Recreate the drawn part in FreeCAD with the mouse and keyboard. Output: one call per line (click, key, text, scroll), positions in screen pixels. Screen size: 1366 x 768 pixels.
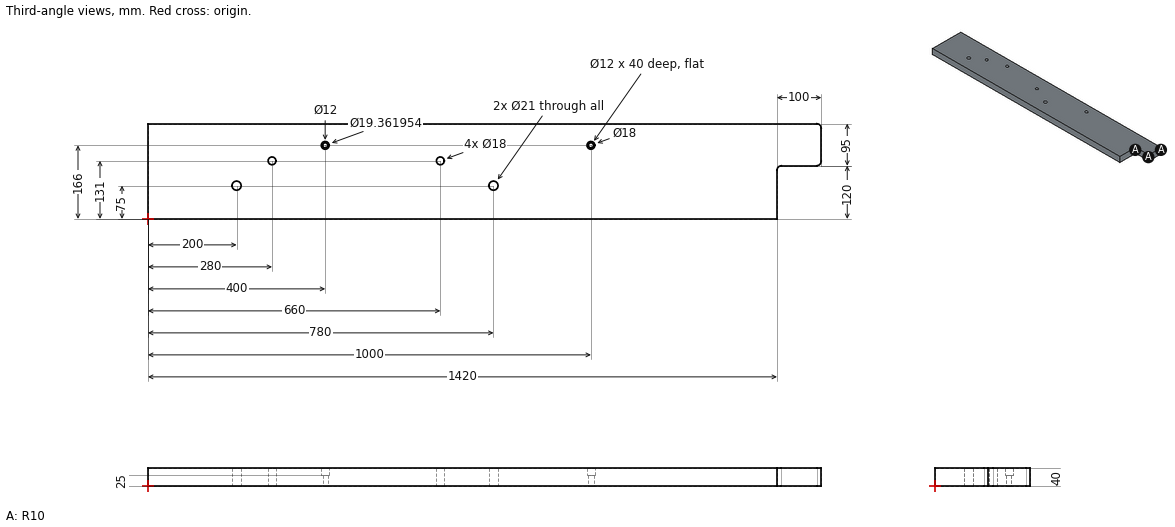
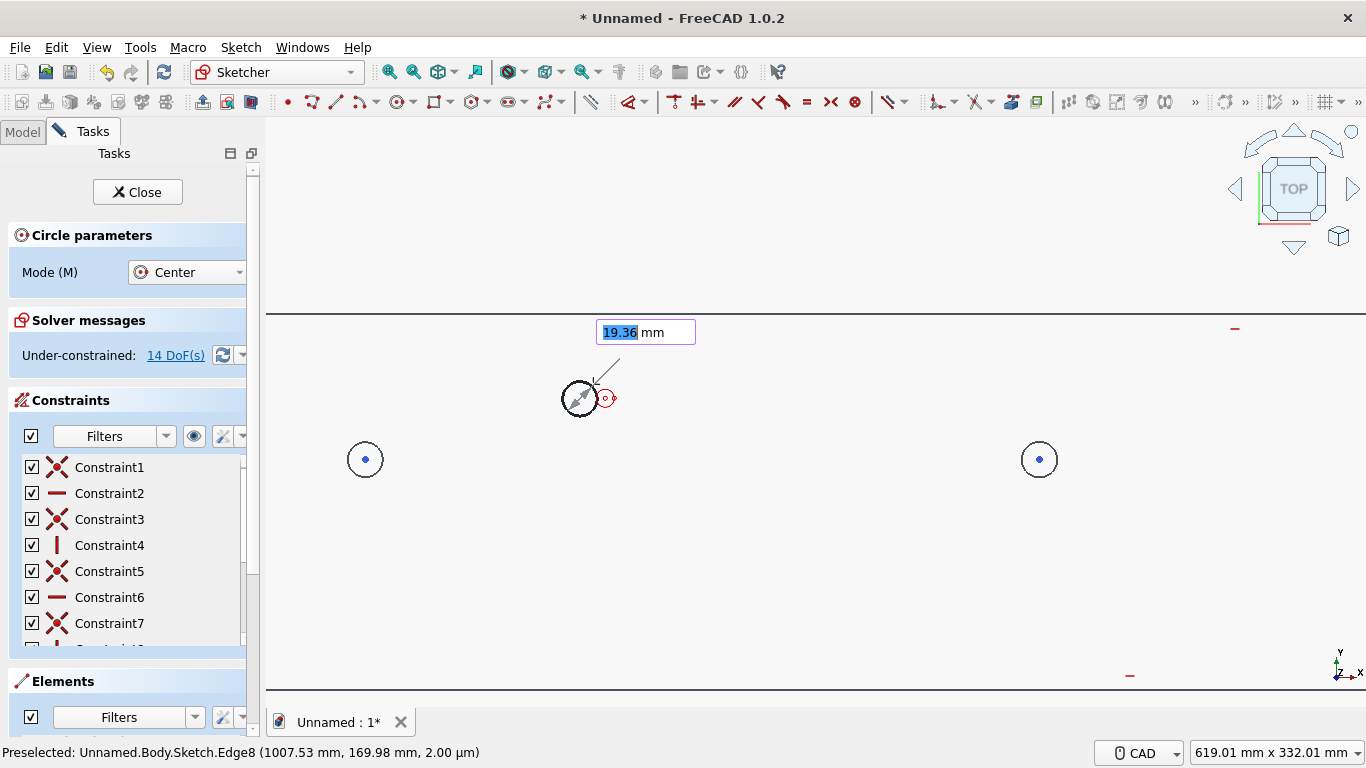
click(590, 384)
key(Escape)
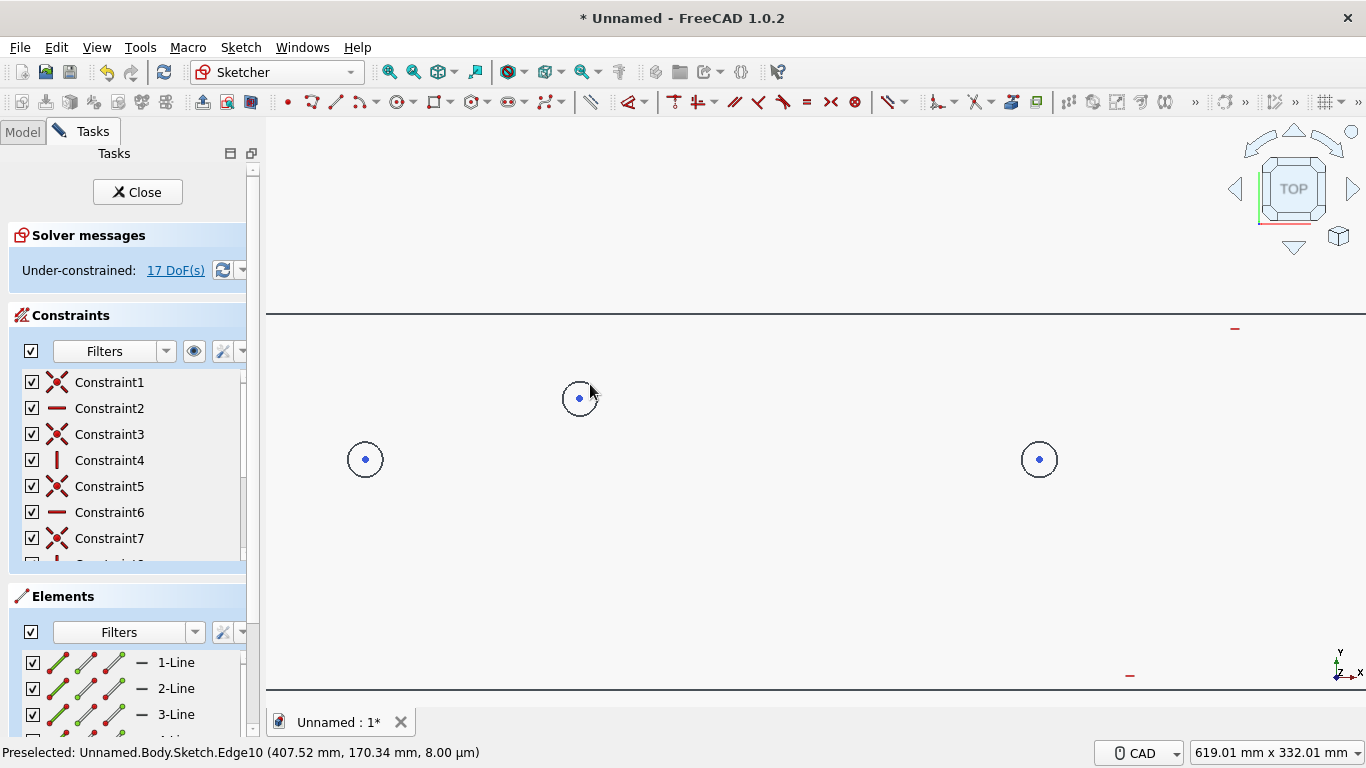
scroll(593, 384, down, 7)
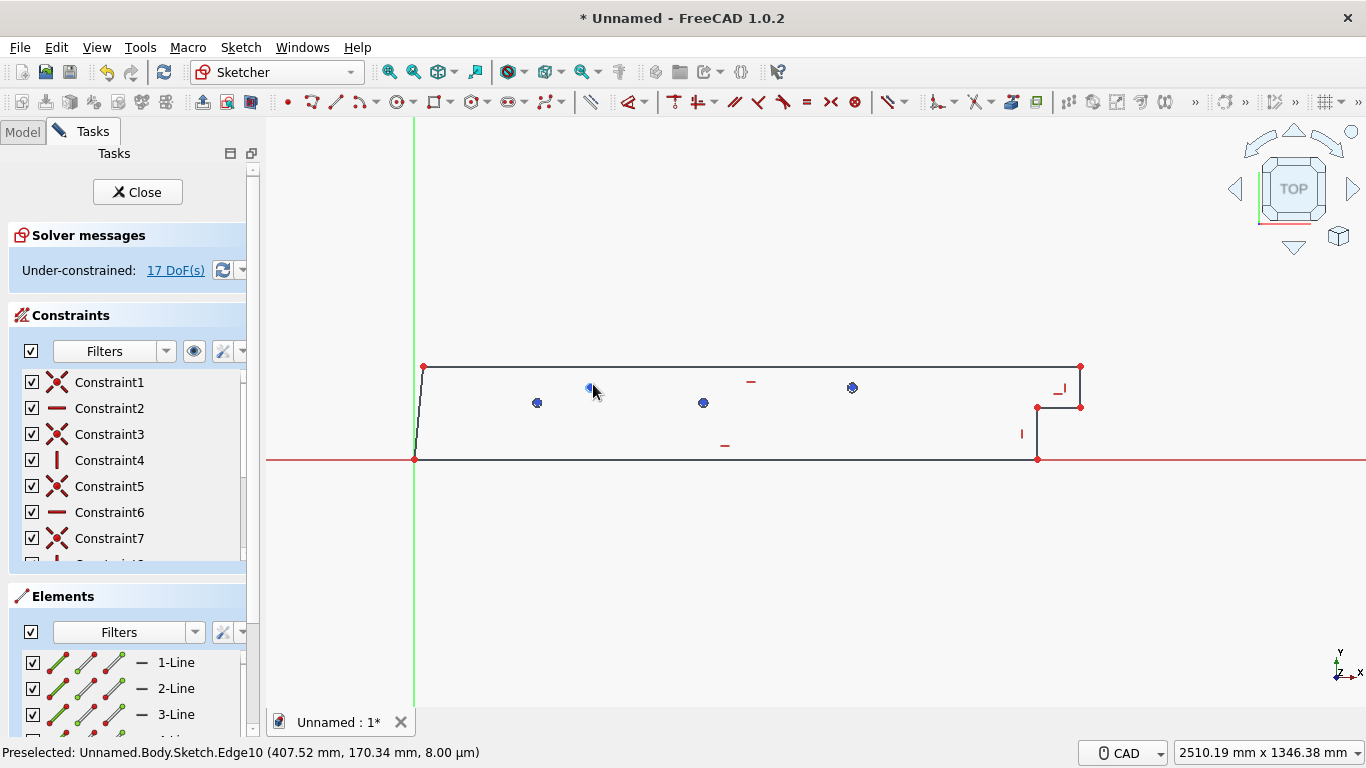
scroll(421, 395, up, 5)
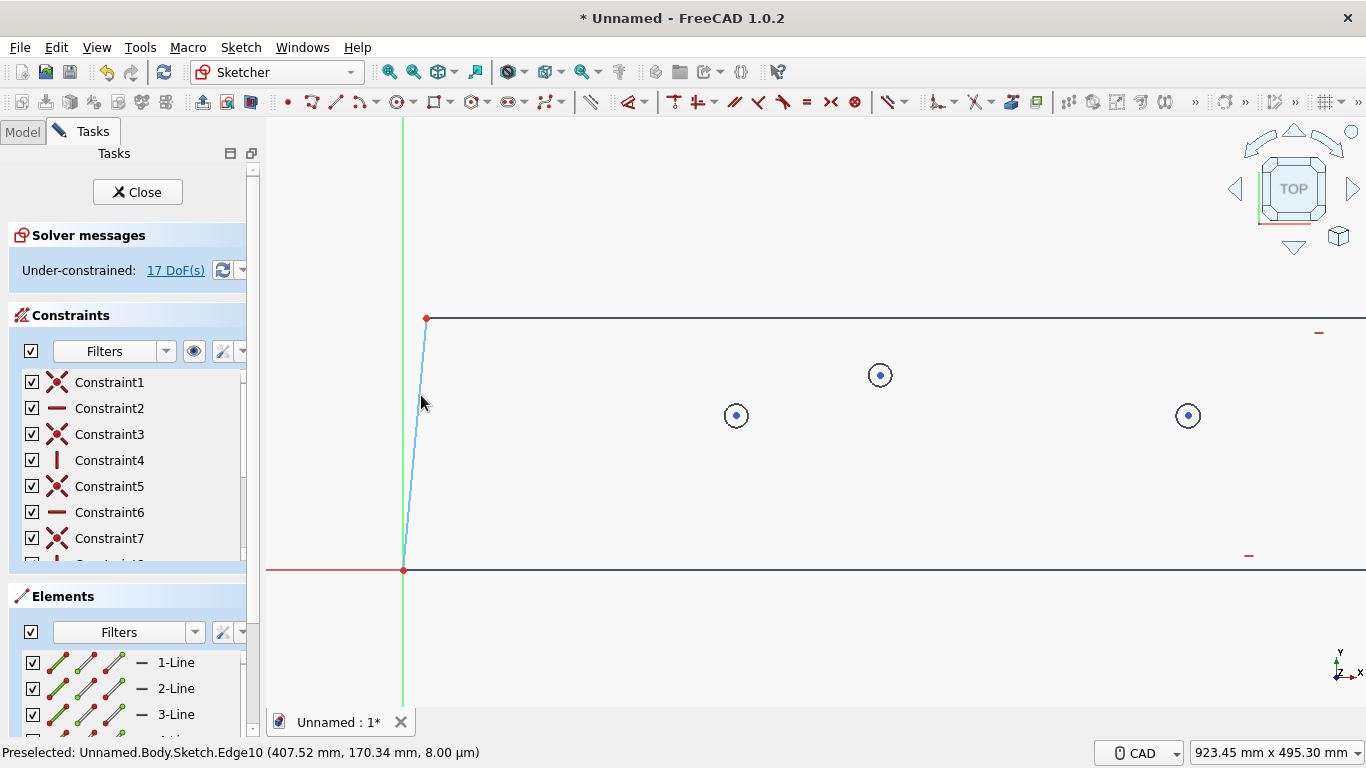
click(420, 394)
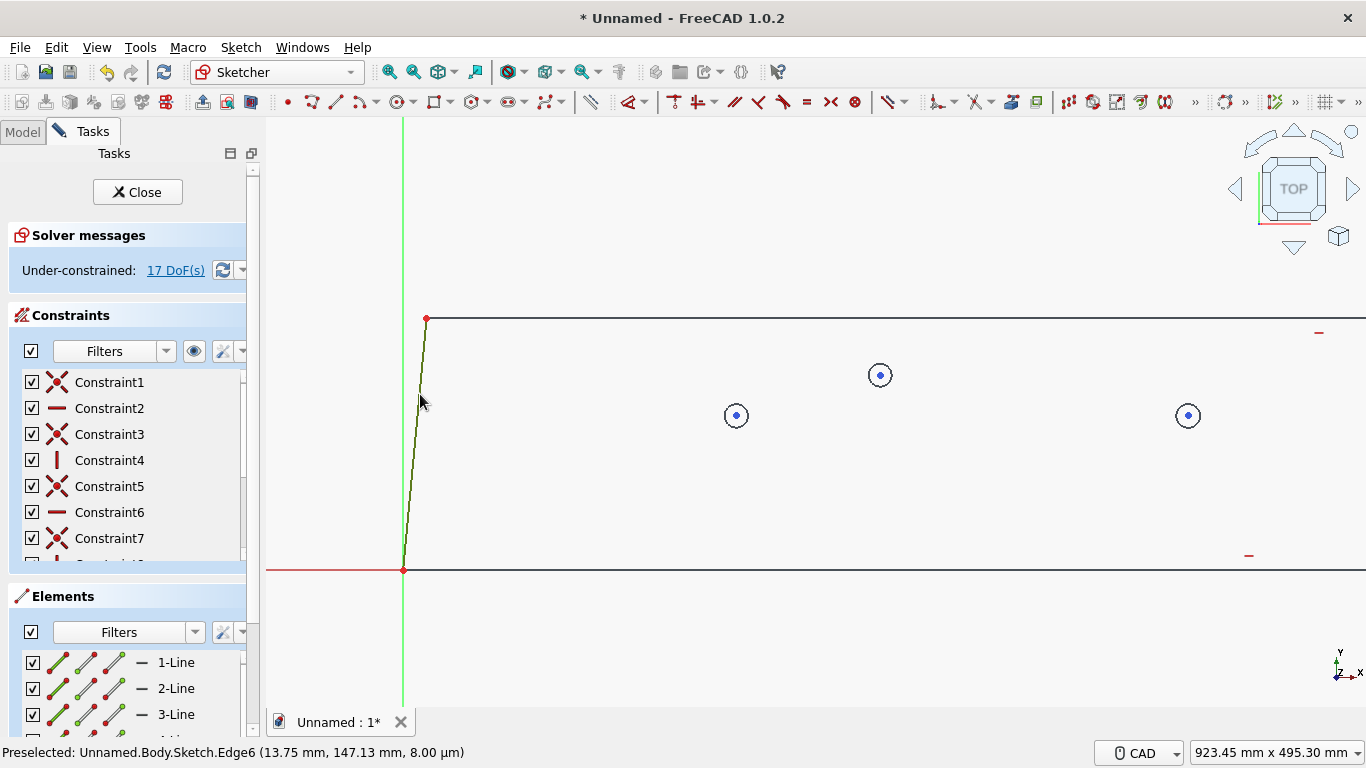
key(v)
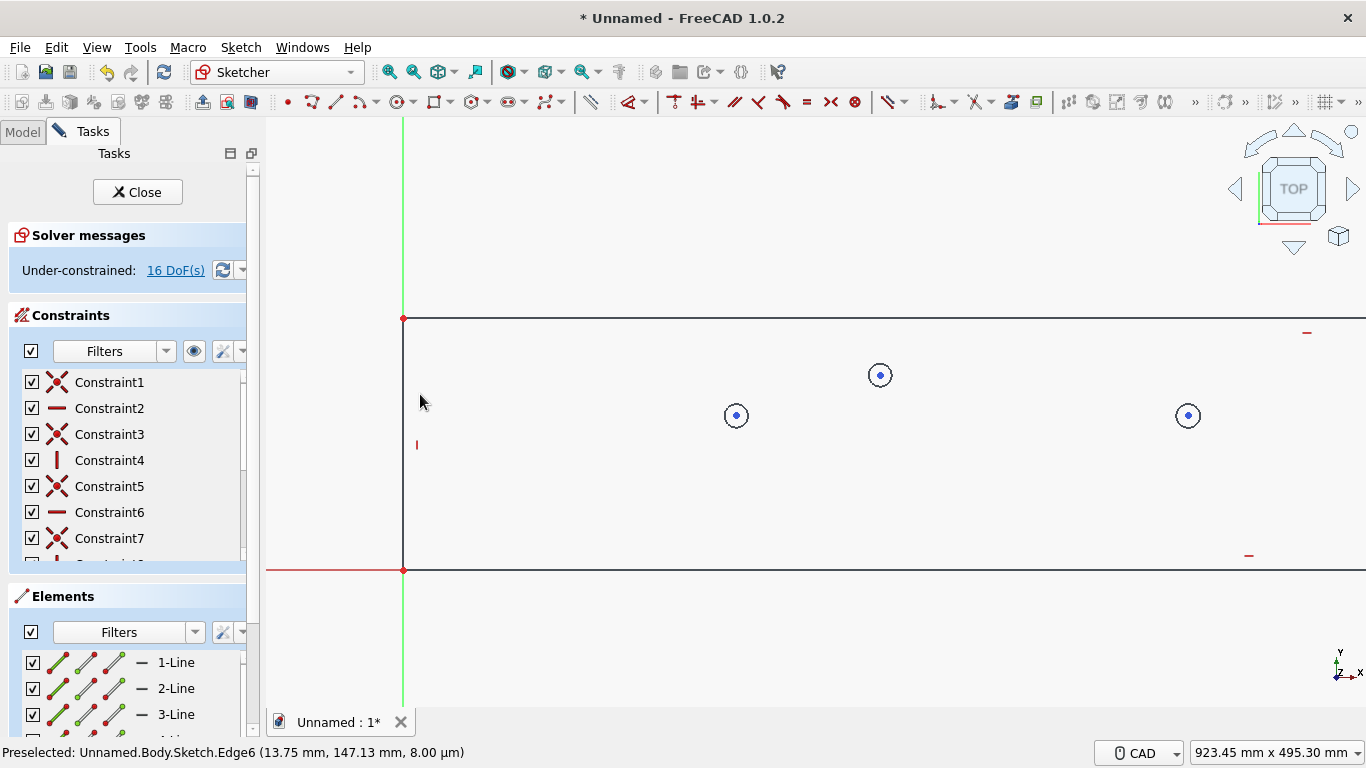
click(1197, 407)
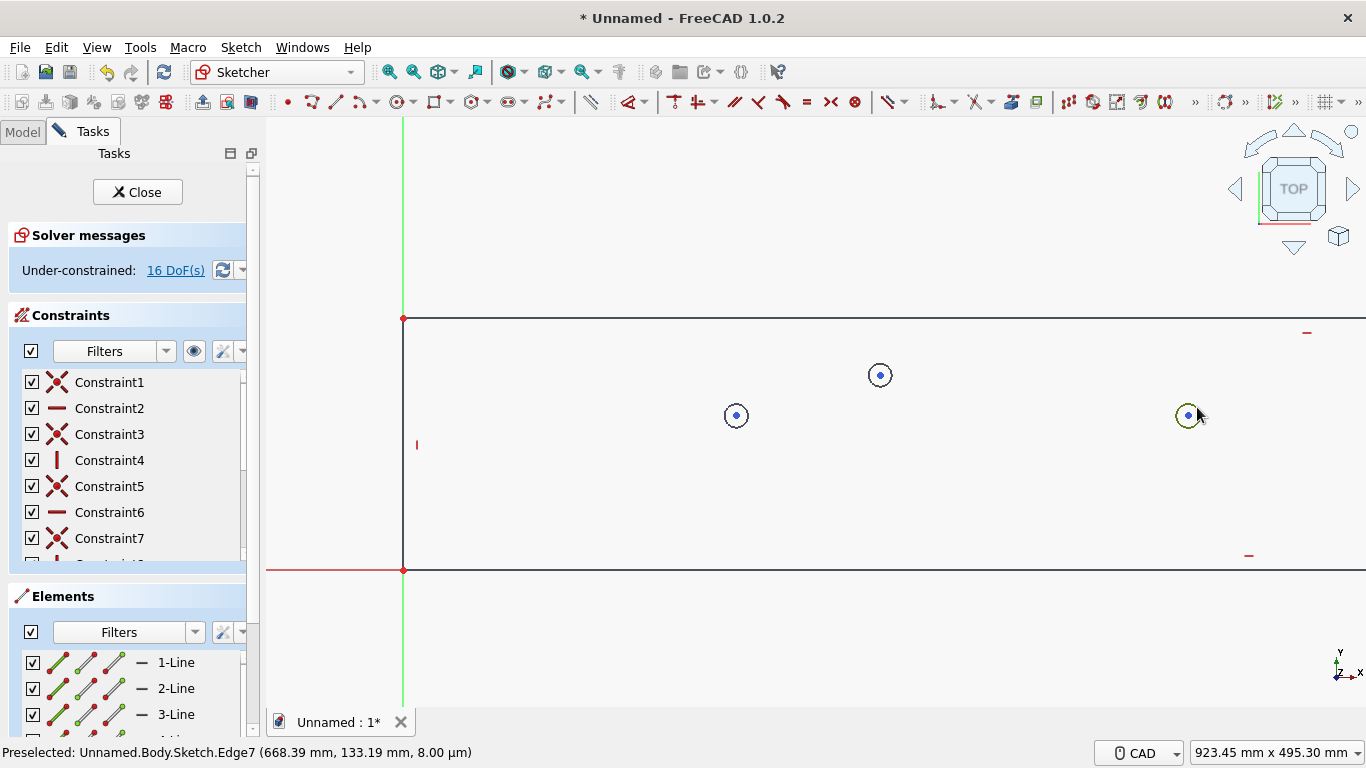
click(745, 408)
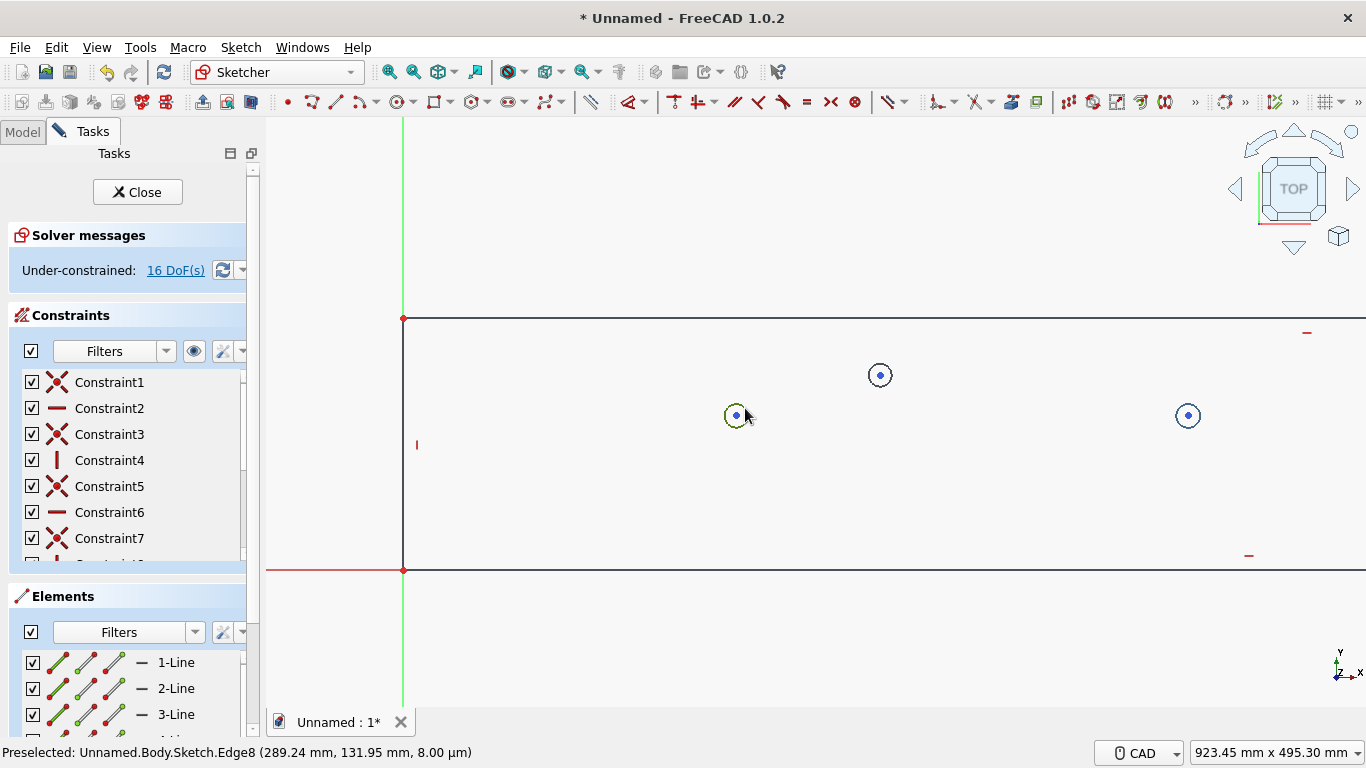
scroll(421, 394, down, 5)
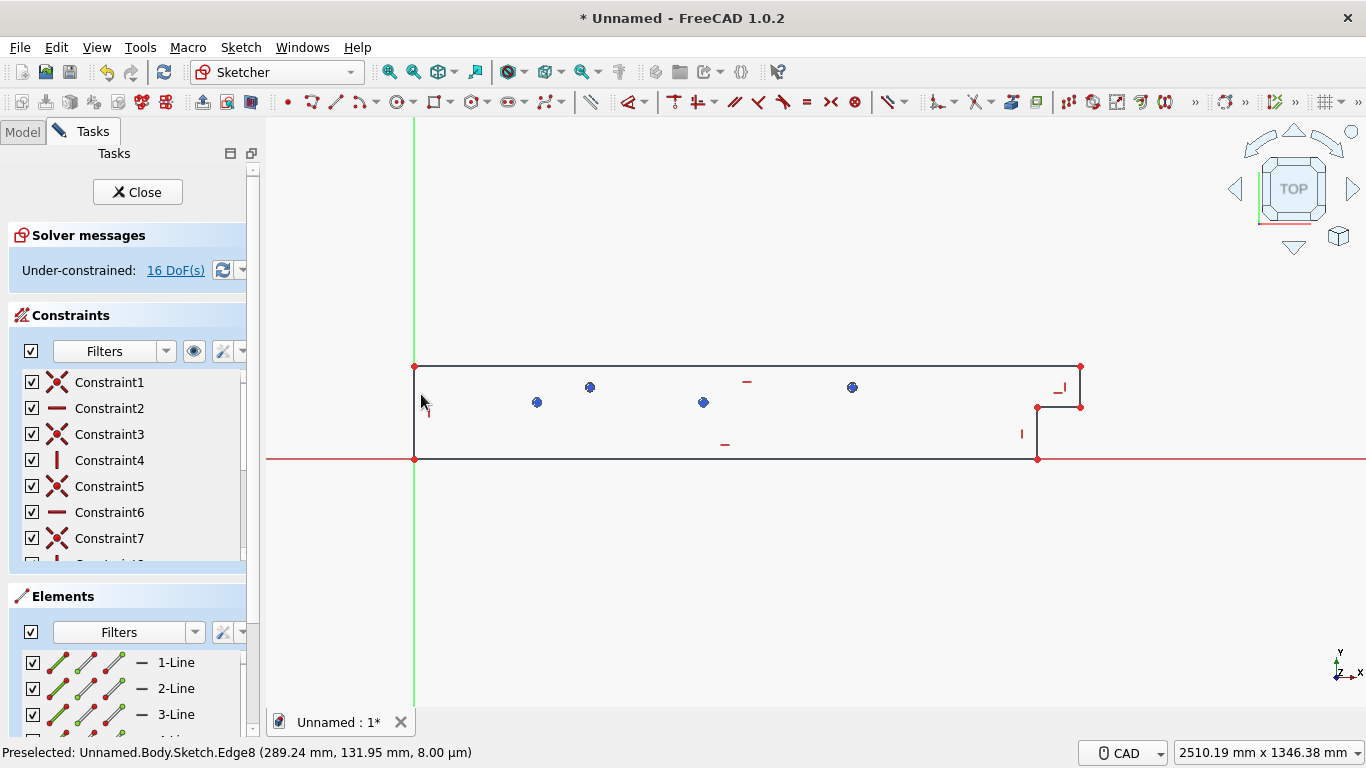
scroll(856, 384, up, 6)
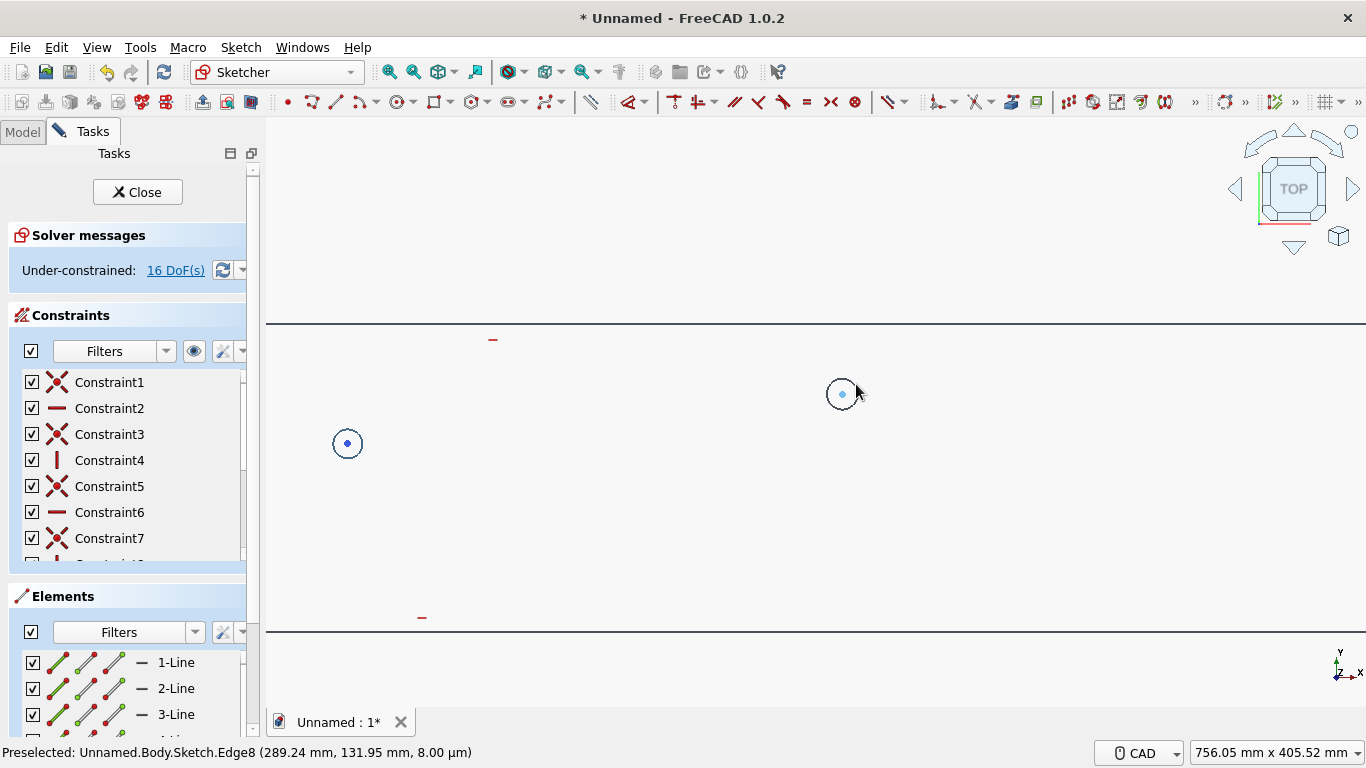
click(853, 383)